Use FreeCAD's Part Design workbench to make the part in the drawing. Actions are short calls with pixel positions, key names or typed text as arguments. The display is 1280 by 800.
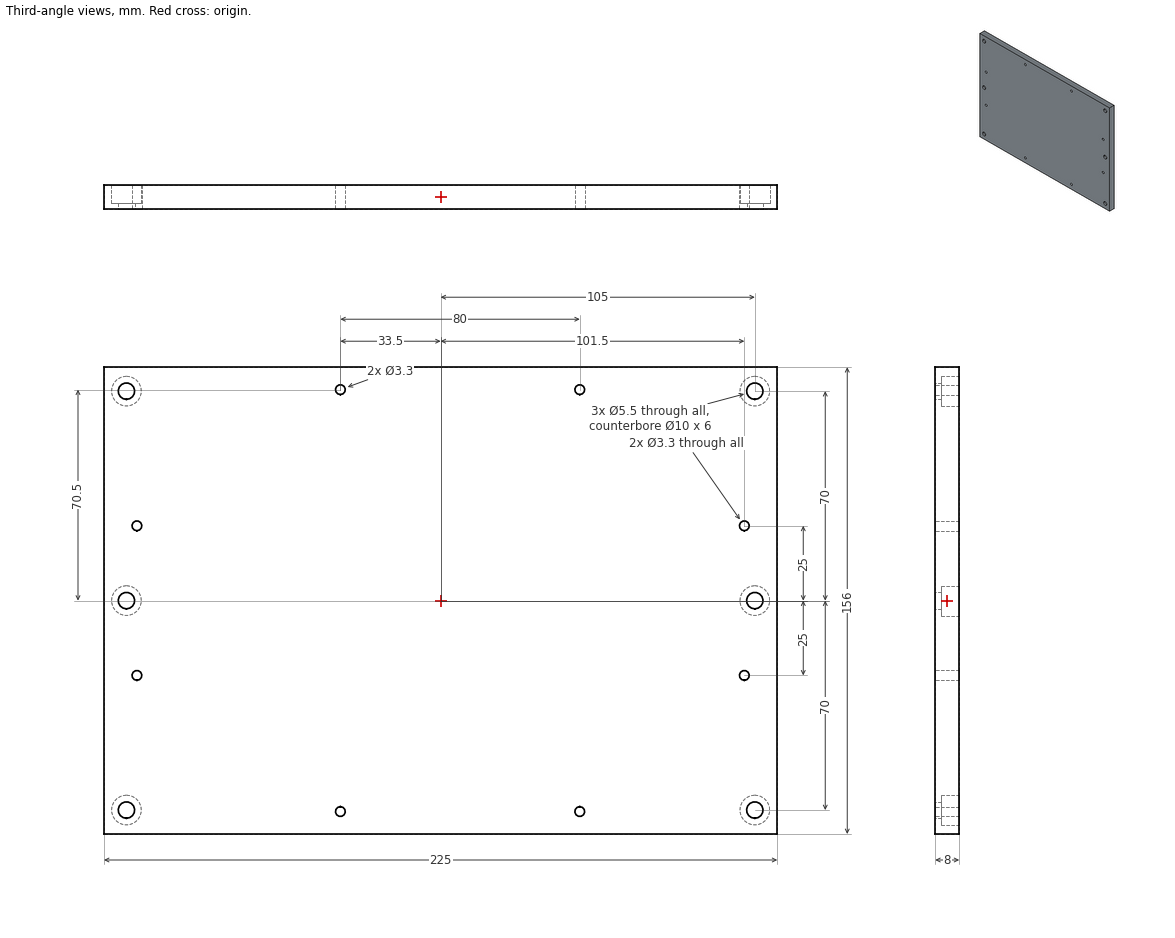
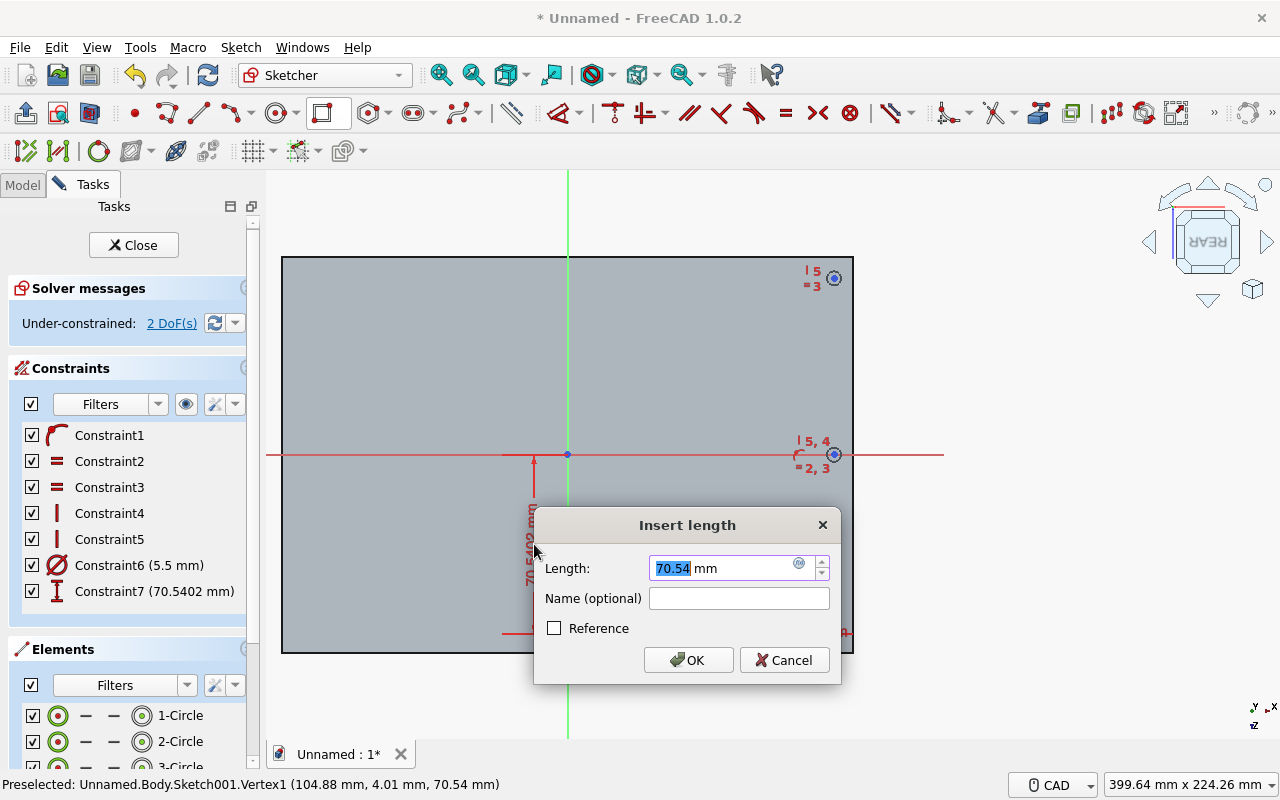
text(70)
key(Return)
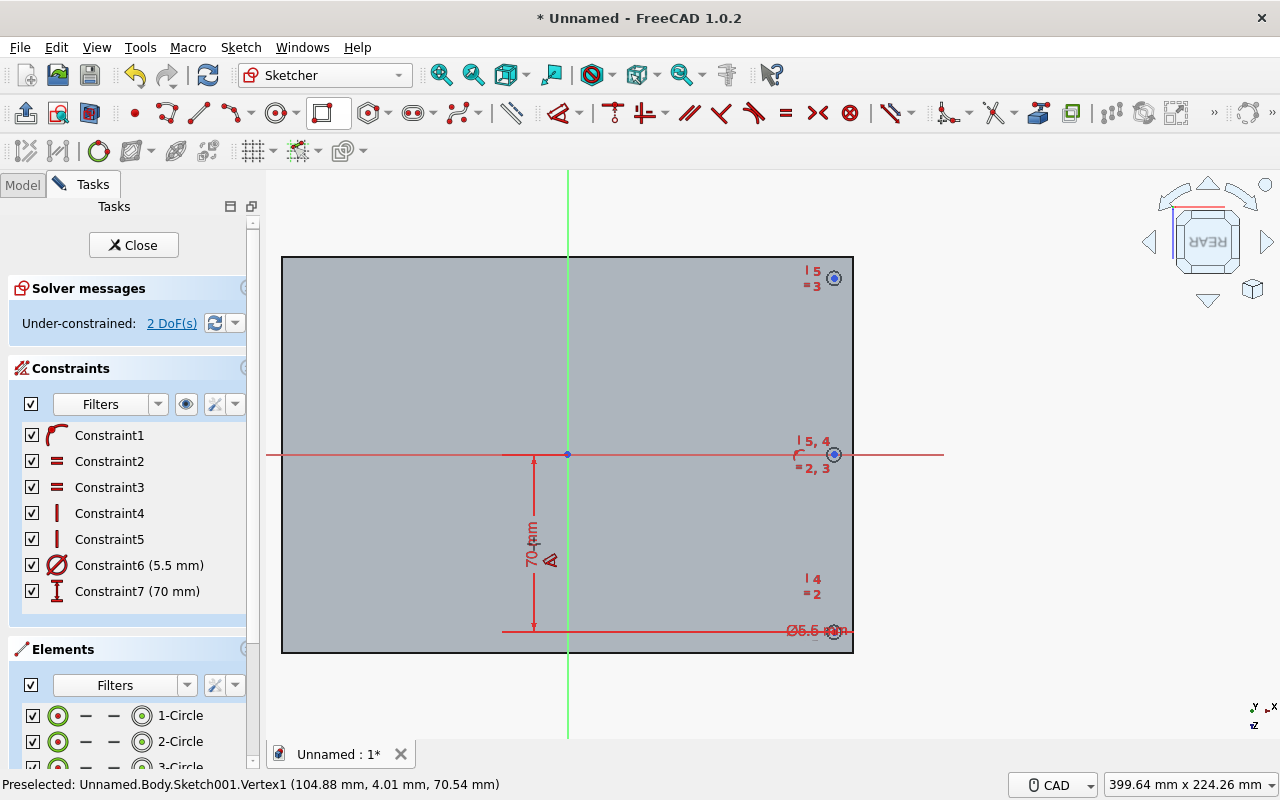
click(834, 278)
click(534, 367)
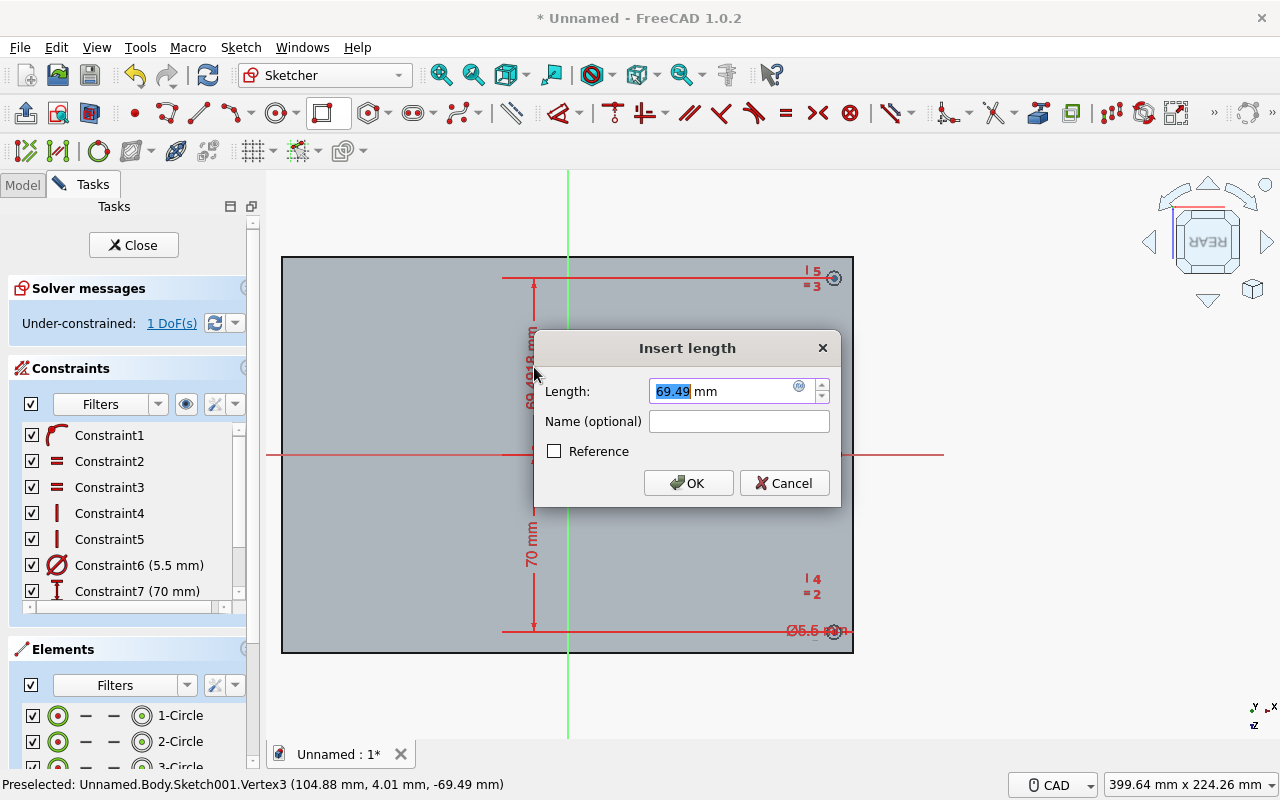
text(70)
key(Return)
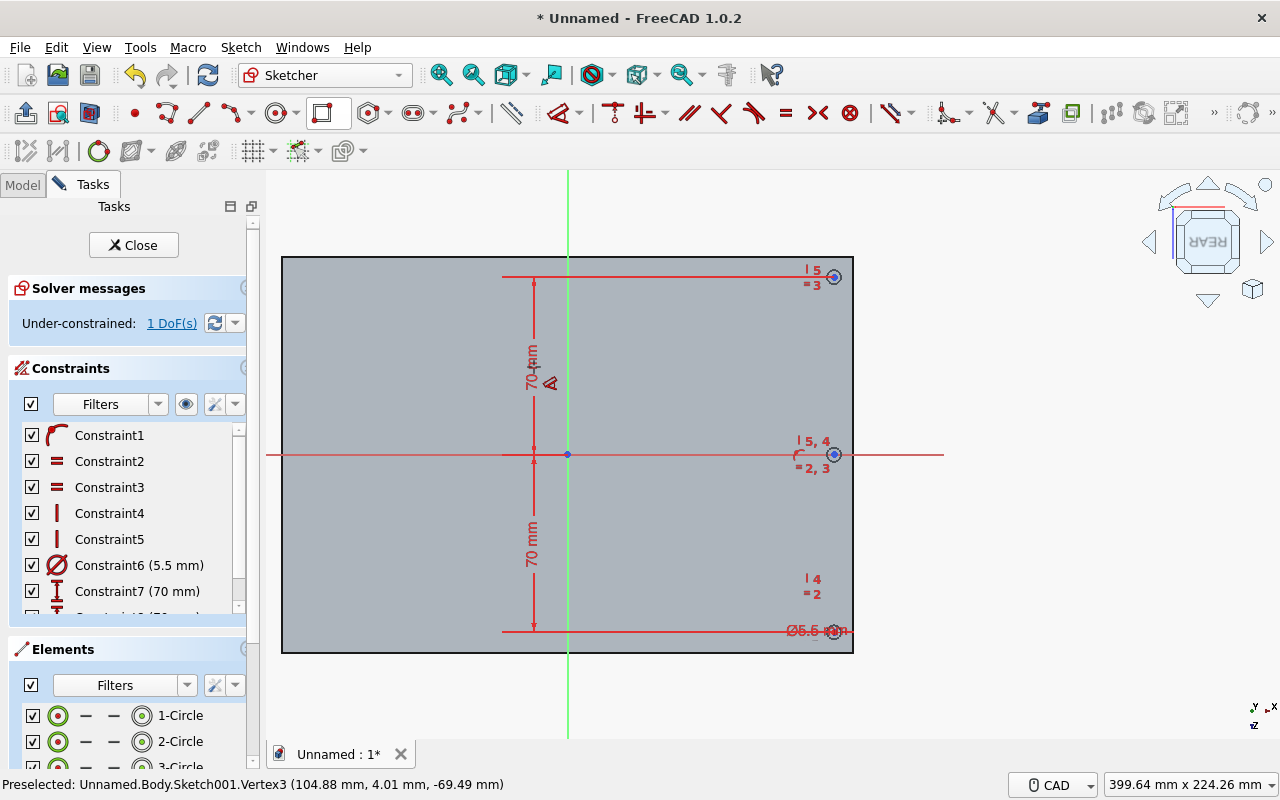
click(834, 632)
click(701, 666)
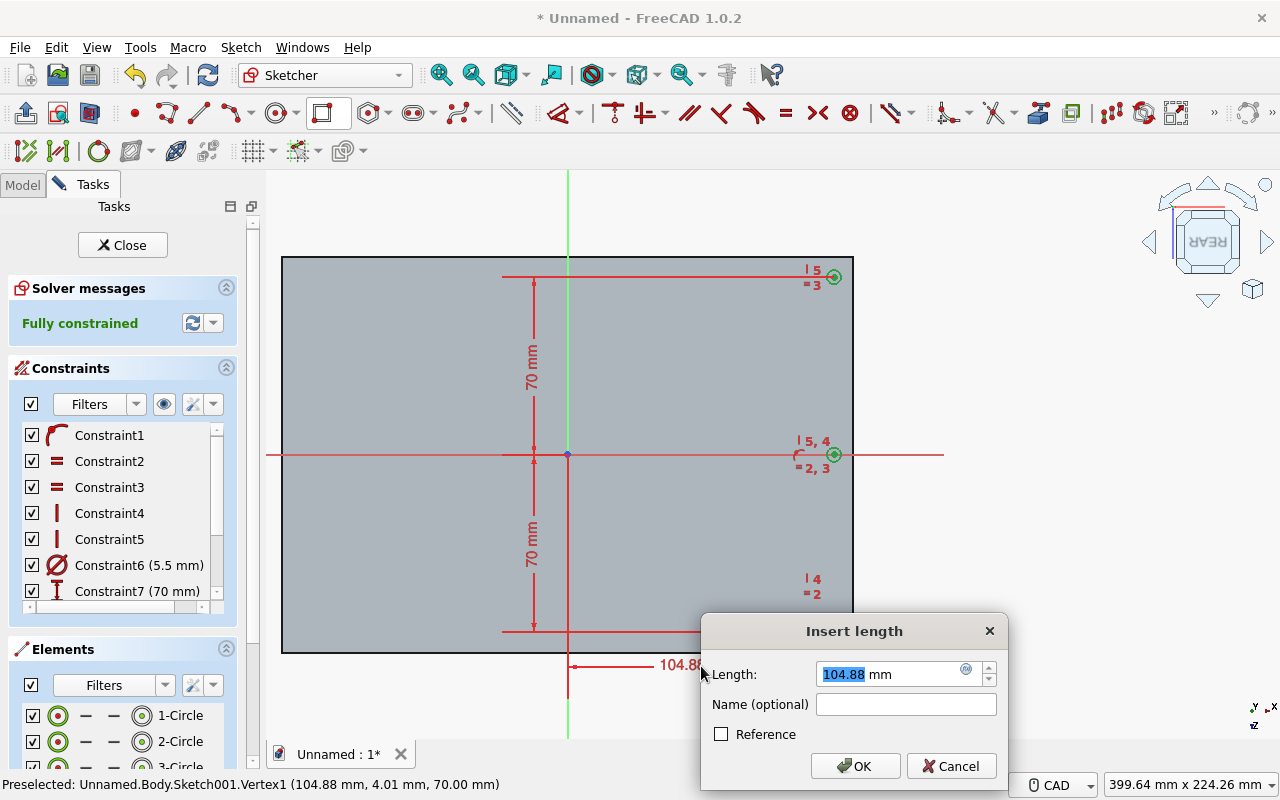
text(105)
key(Return)
key(Escape)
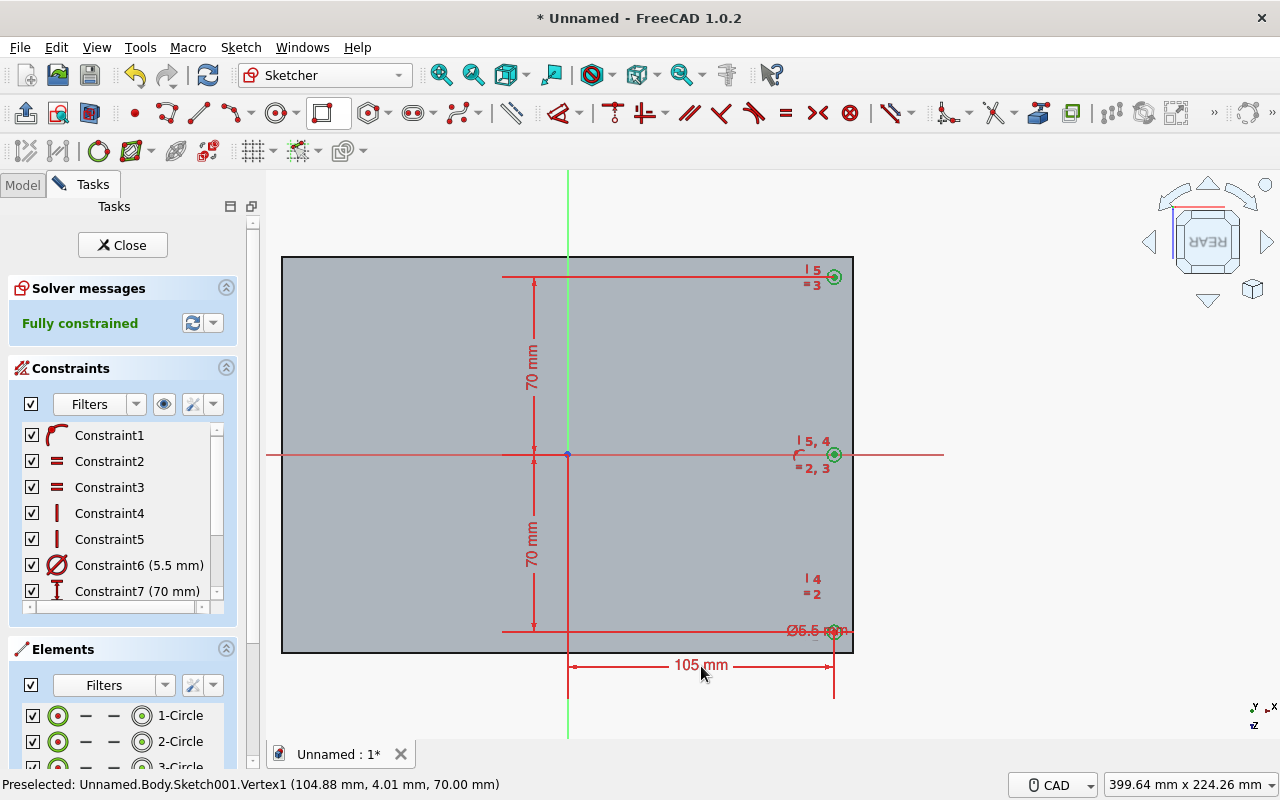
click(123, 245)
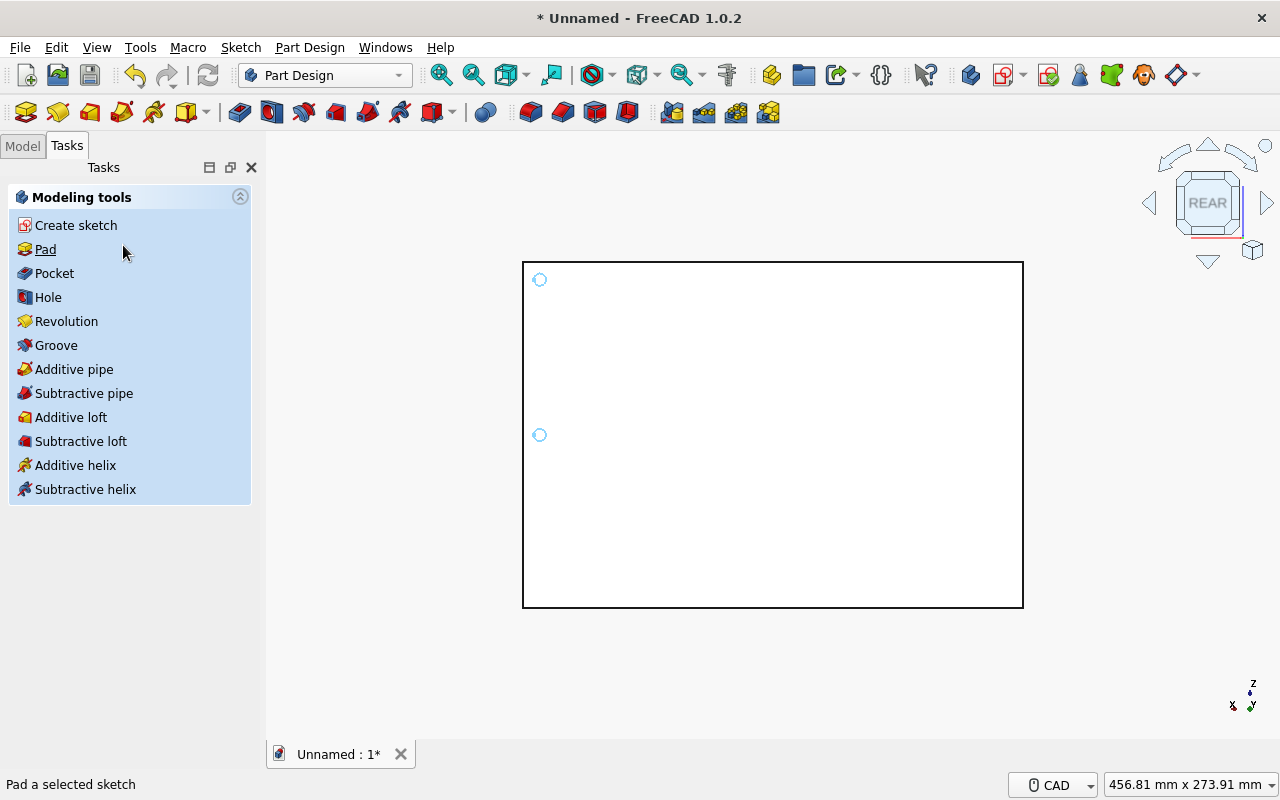
click(272, 112)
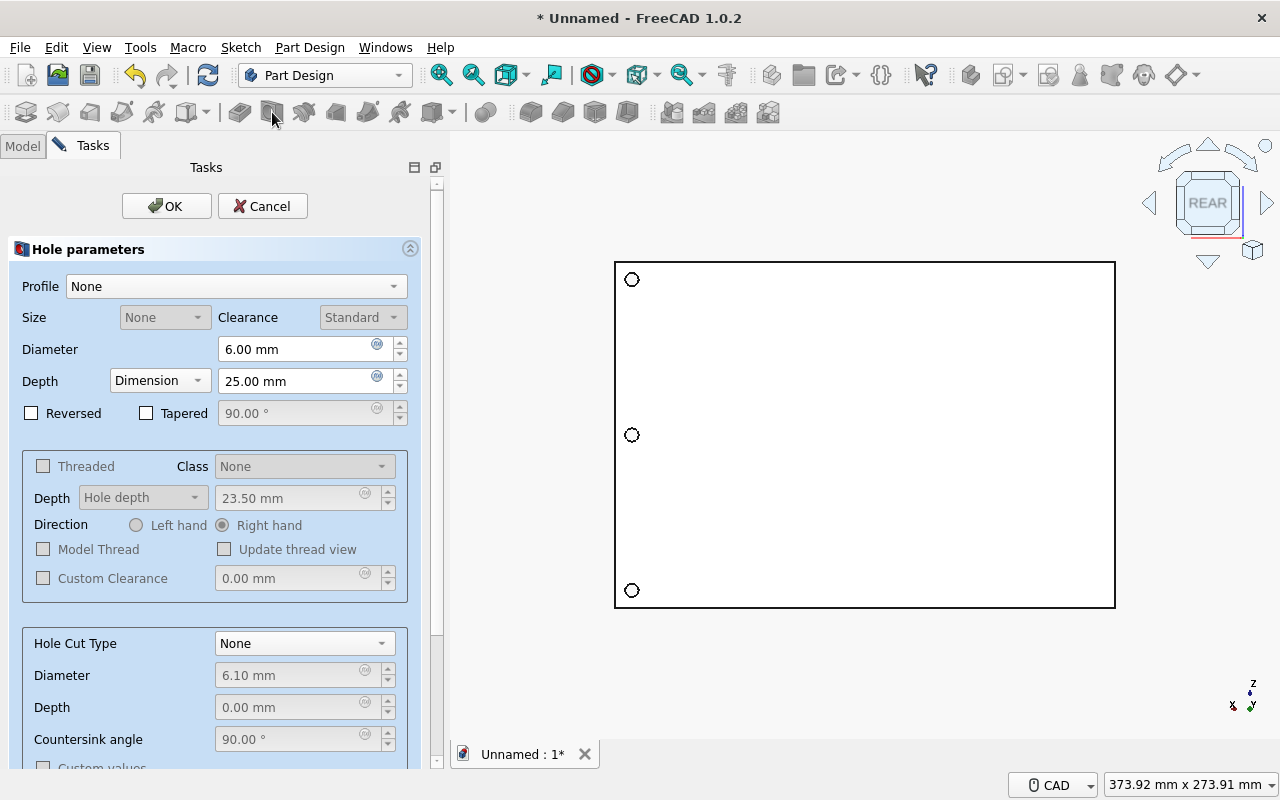
triple_click(305, 349)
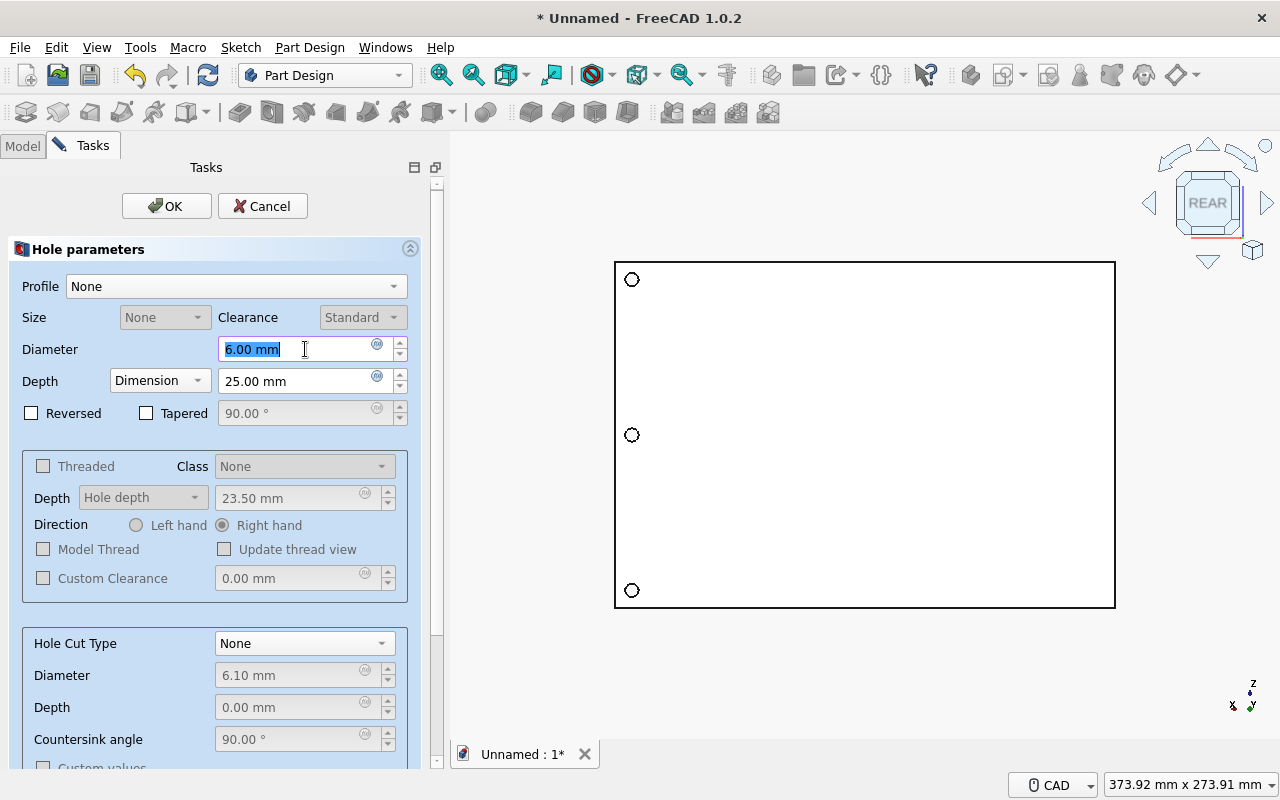
text(5.5)
key(Tab)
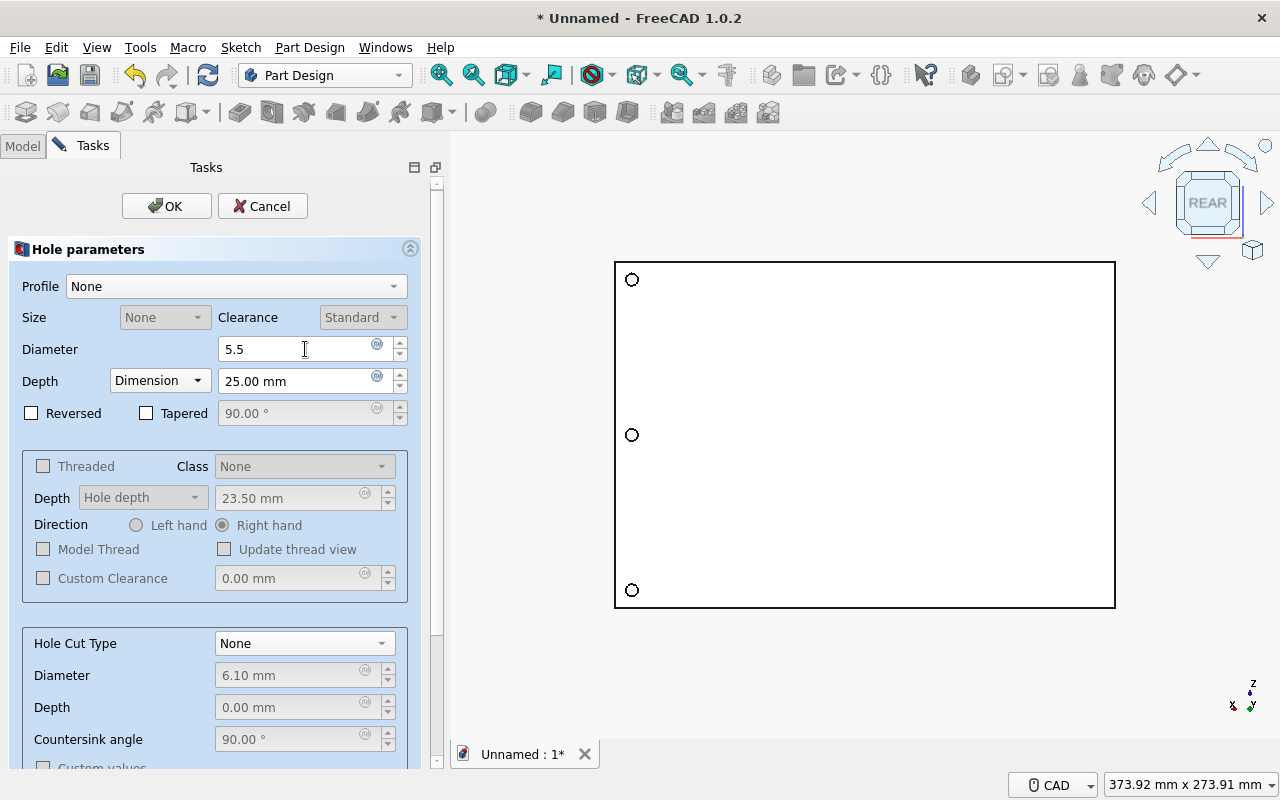
click(161, 380)